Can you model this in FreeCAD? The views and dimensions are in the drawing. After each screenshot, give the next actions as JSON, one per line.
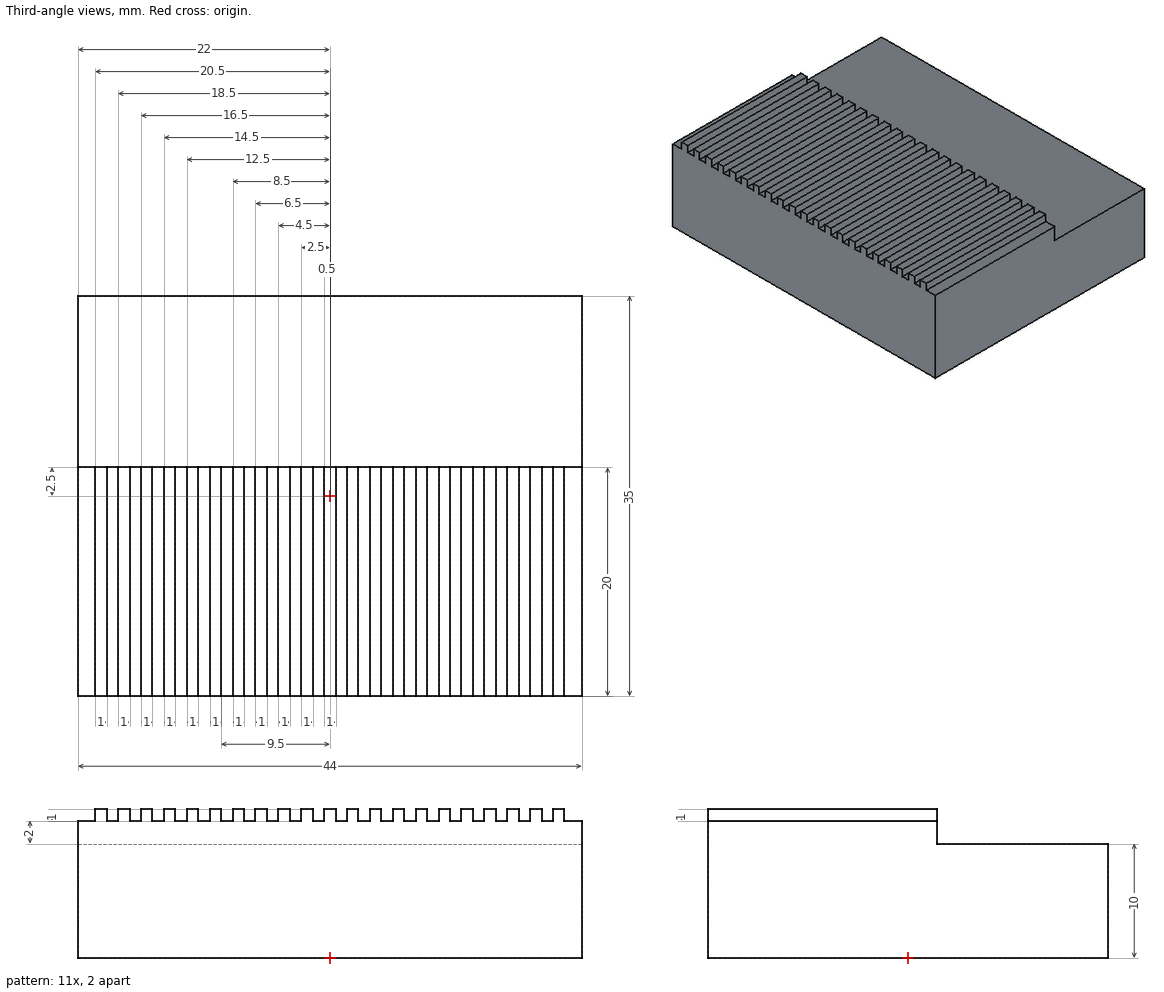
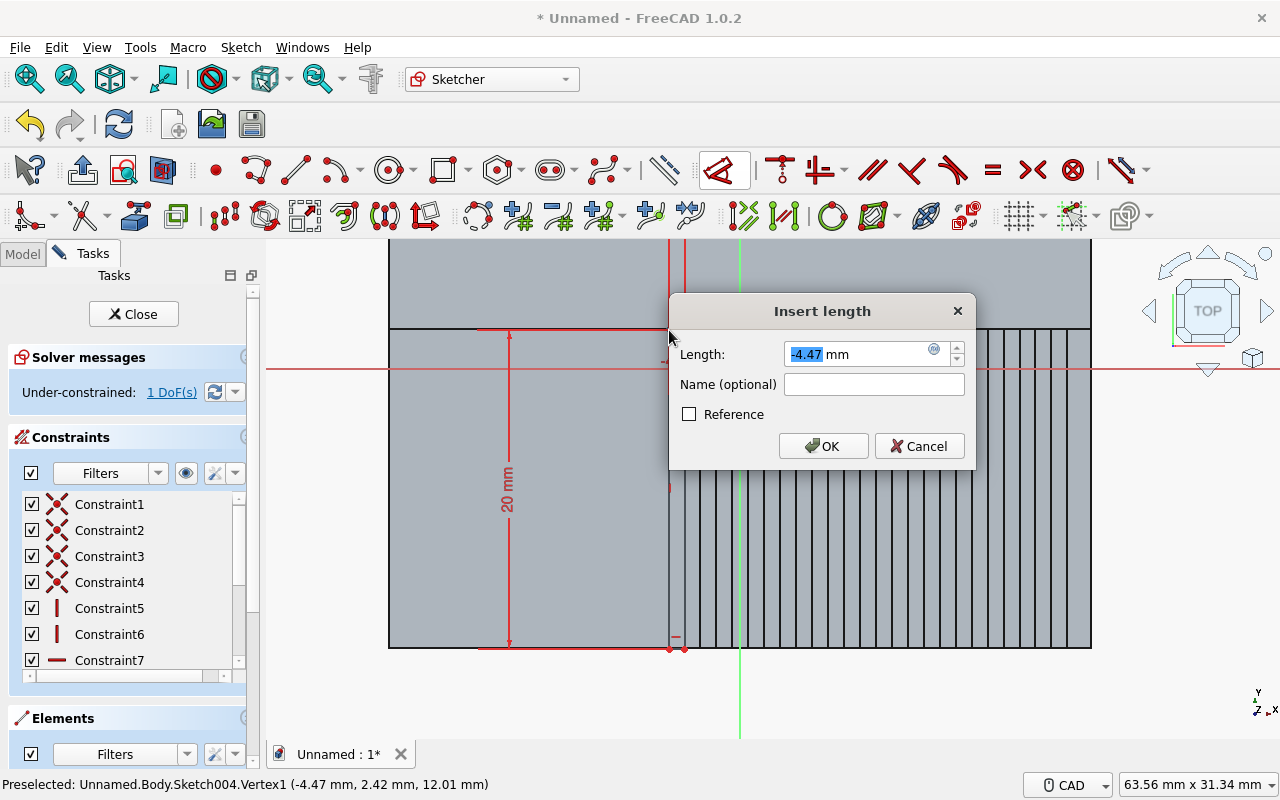
{"action": "type", "text": "-4.5"}
{"action": "key", "text": "Return"}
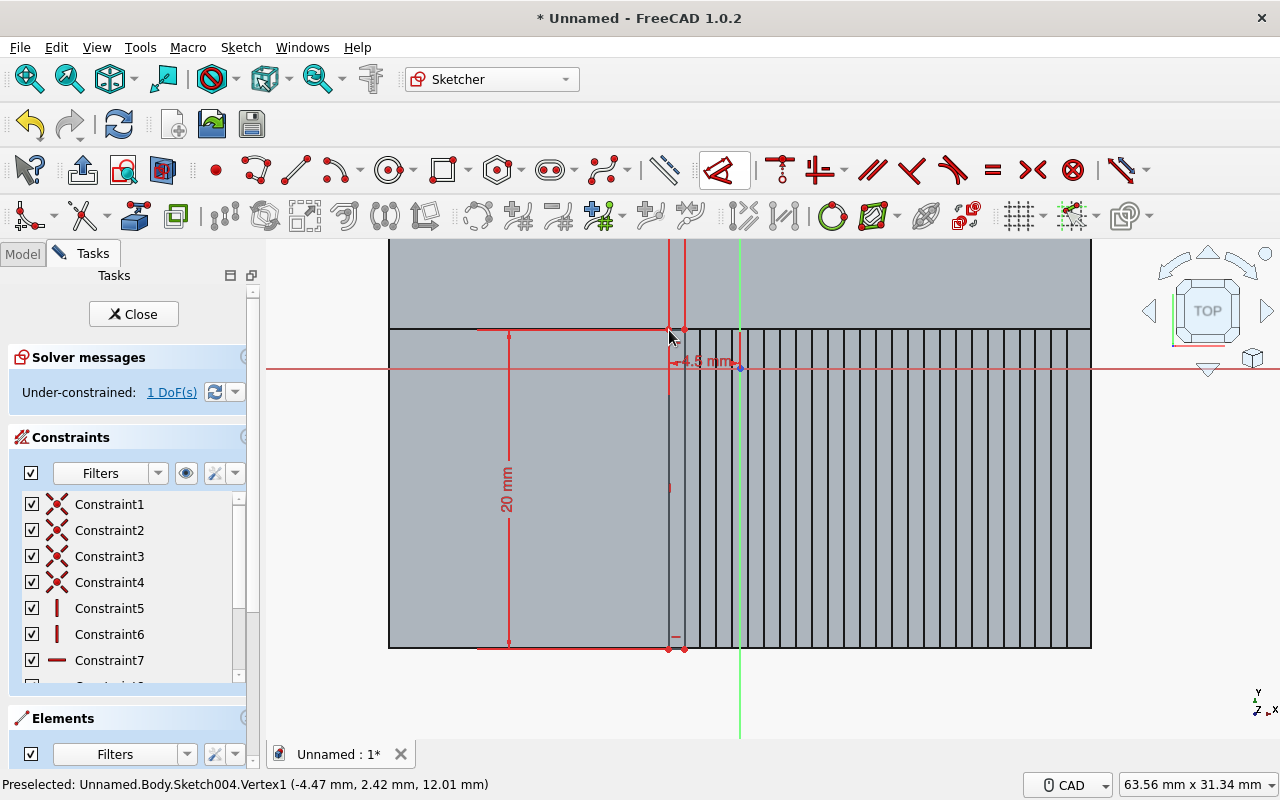
{"action": "left_click", "coordinate": [669, 330]}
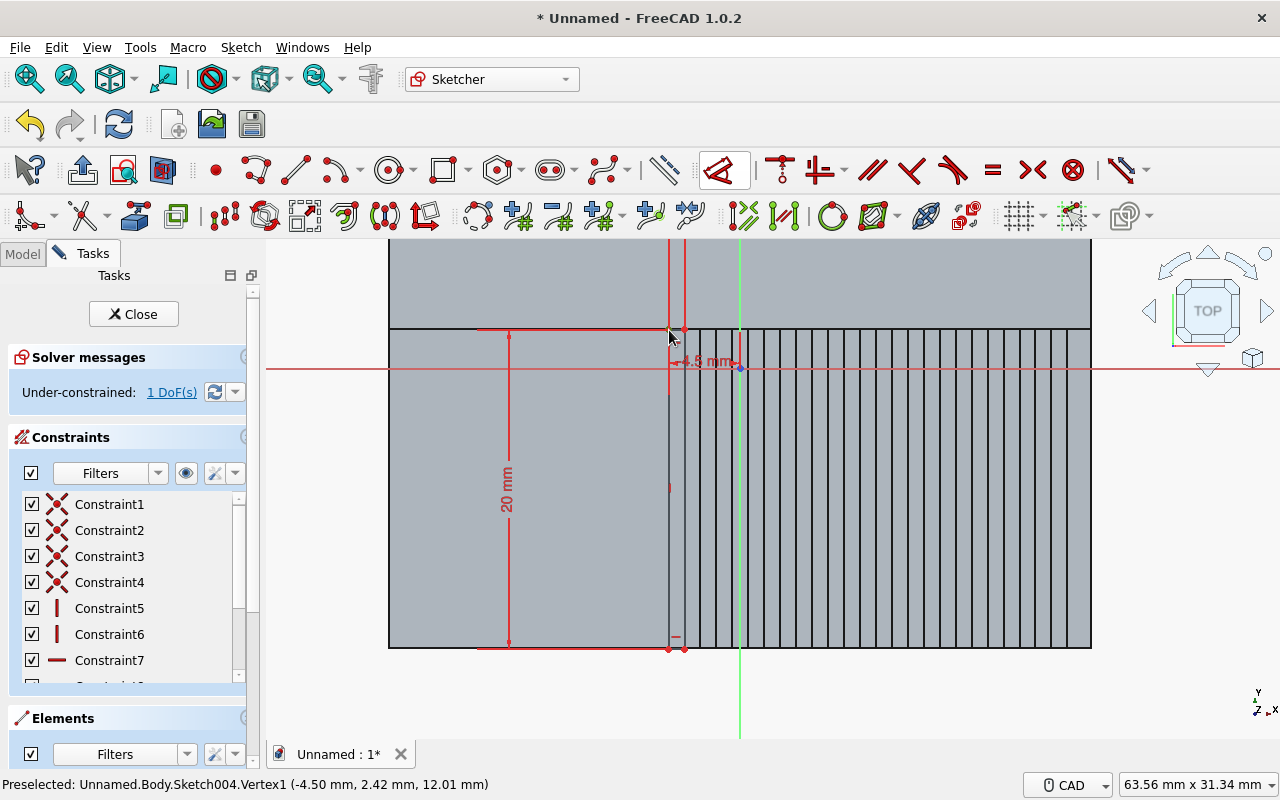
{"action": "key", "text": "i"}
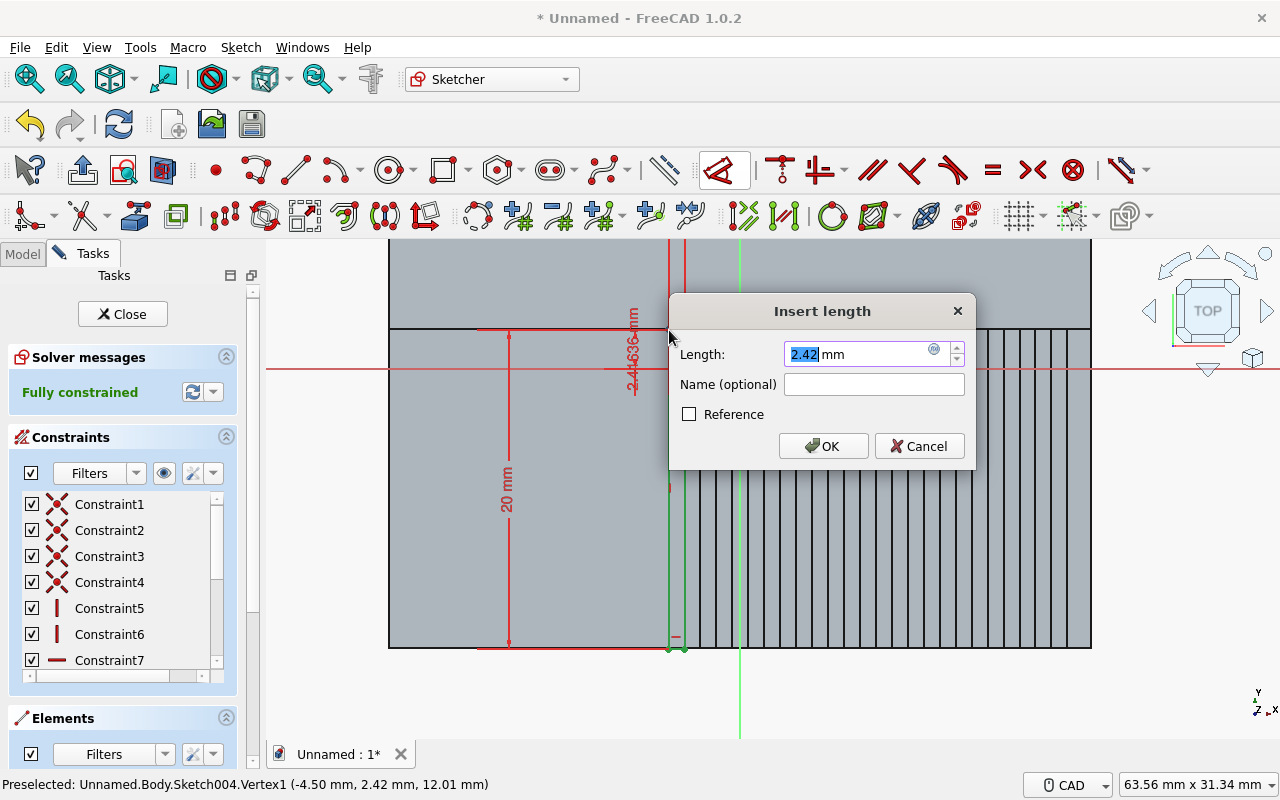
{"action": "type", "text": "2.5"}
{"action": "key", "text": "Return"}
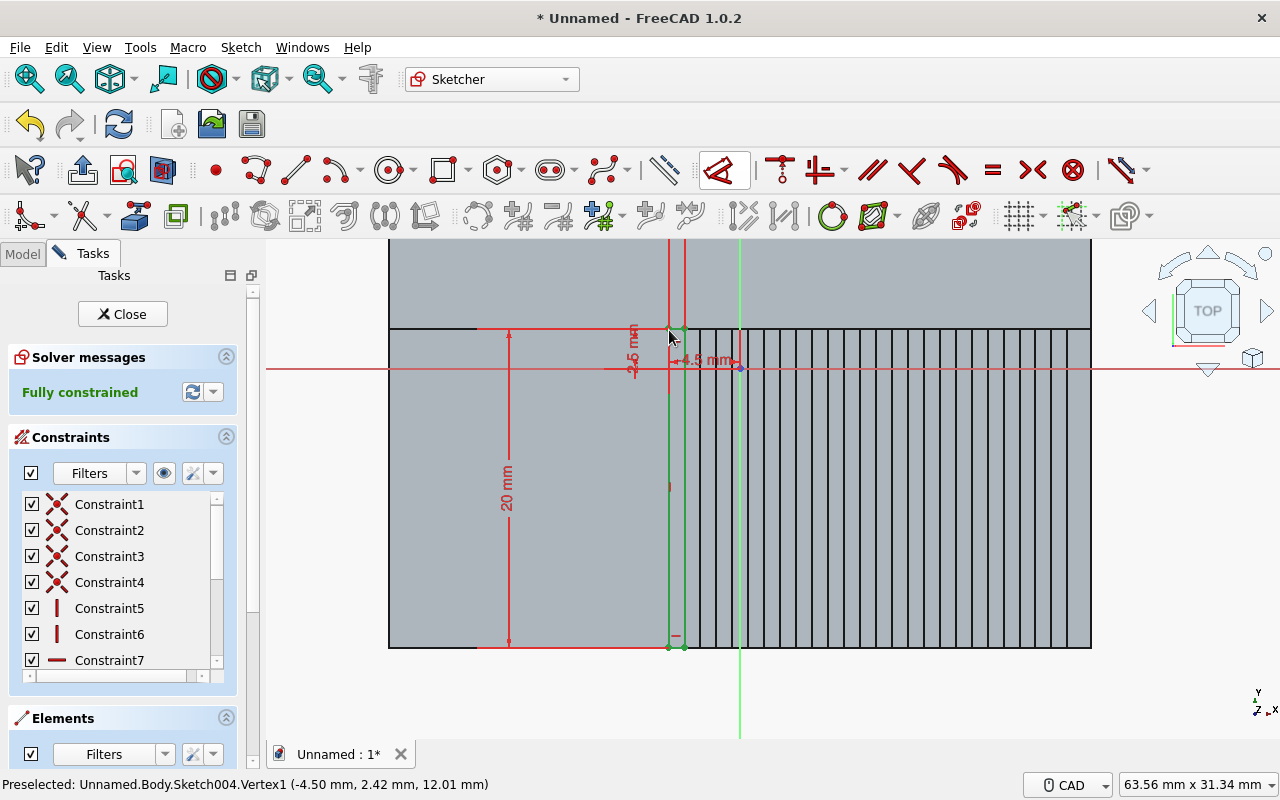
{"action": "left_click", "coordinate": [123, 314]}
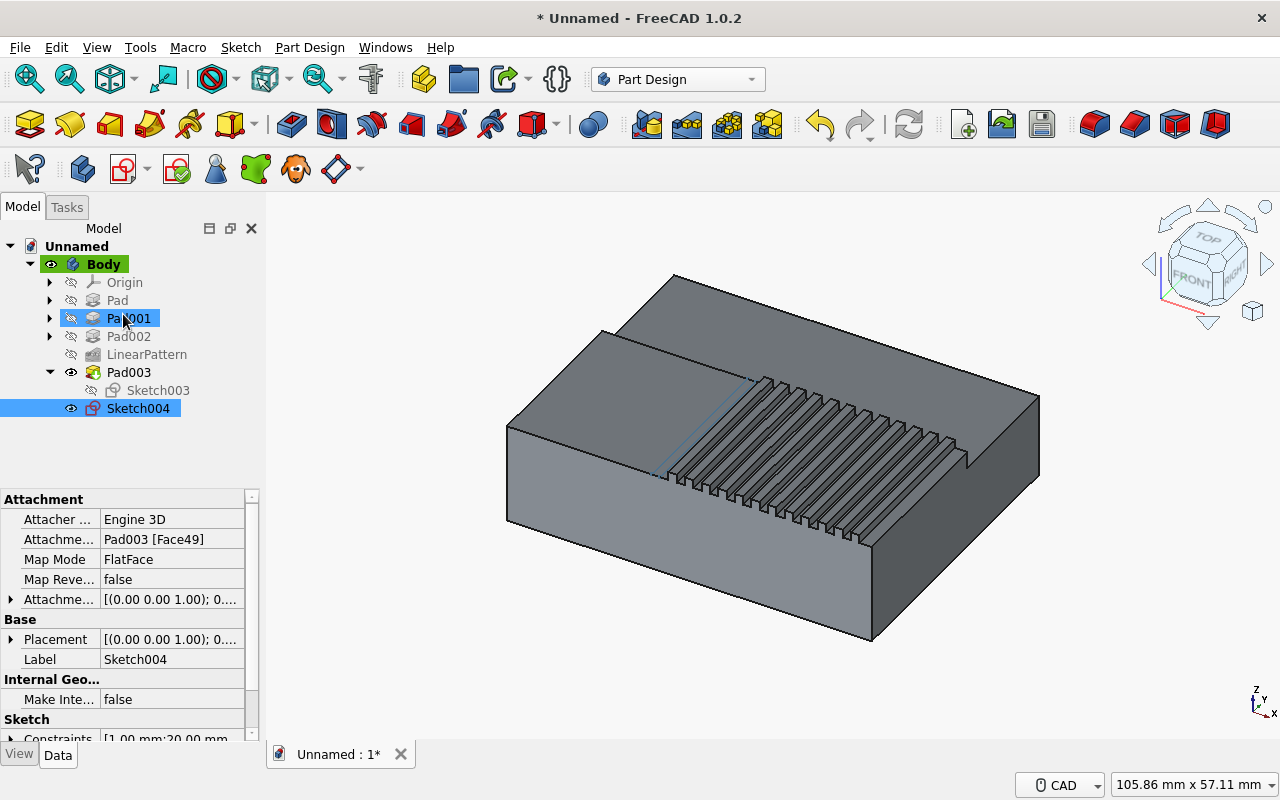
{"action": "left_click", "coordinate": [30, 124]}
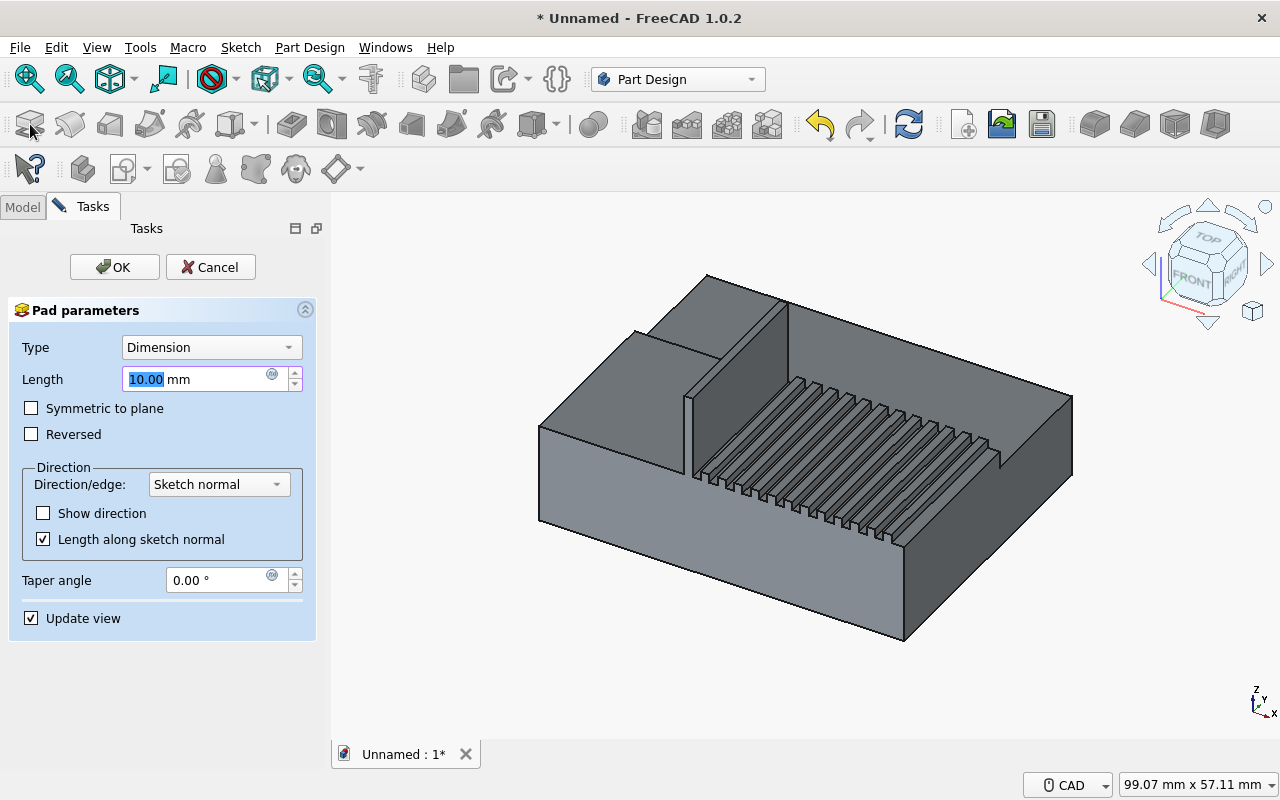
{"action": "type", "text": "1"}
{"action": "key", "text": "Tab"}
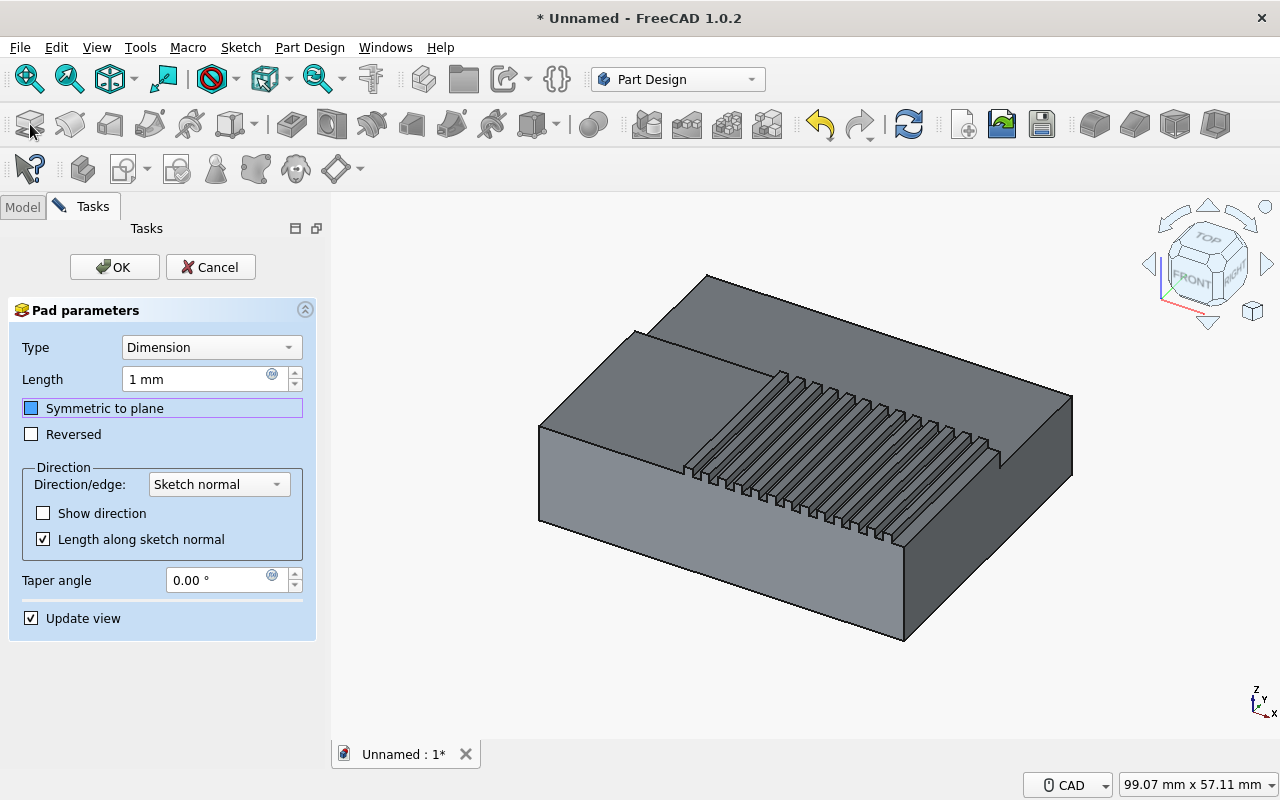
{"action": "left_click", "coordinate": [115, 267]}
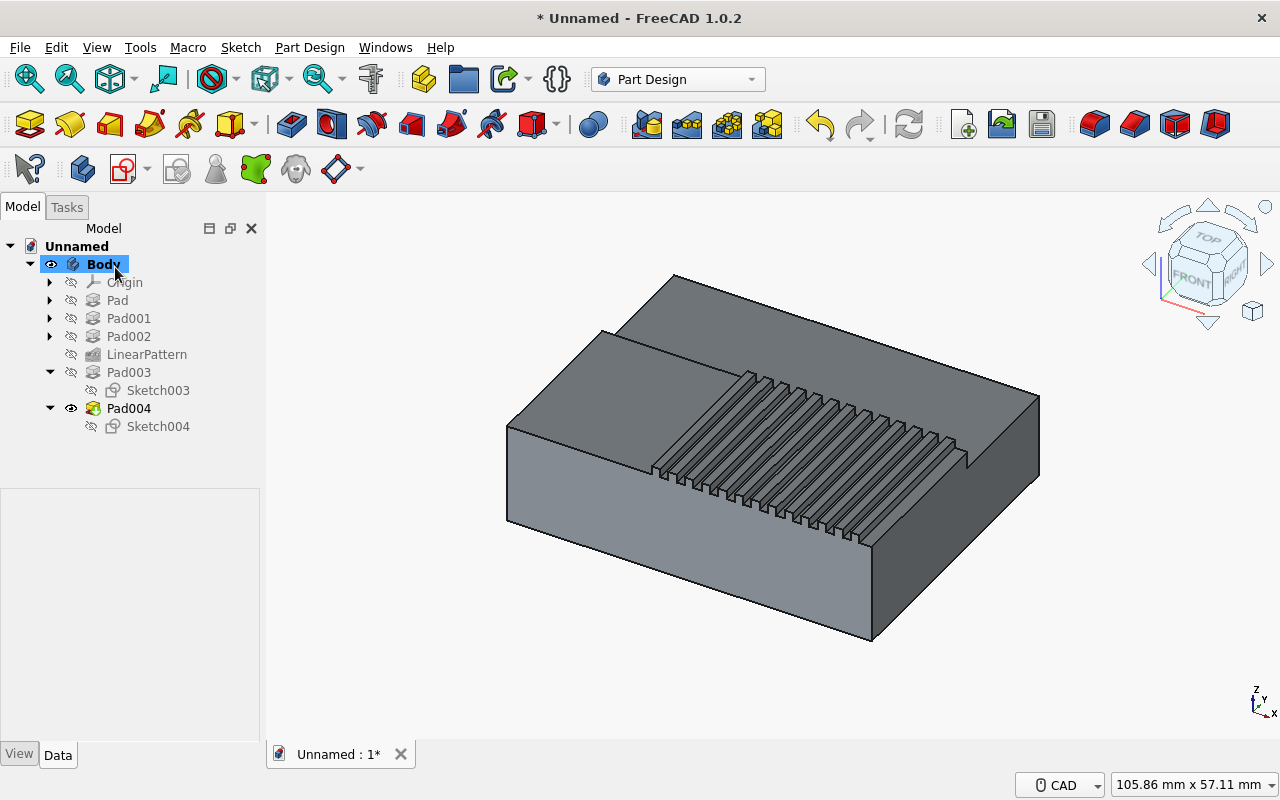
{"action": "left_click", "coordinate": [627, 402]}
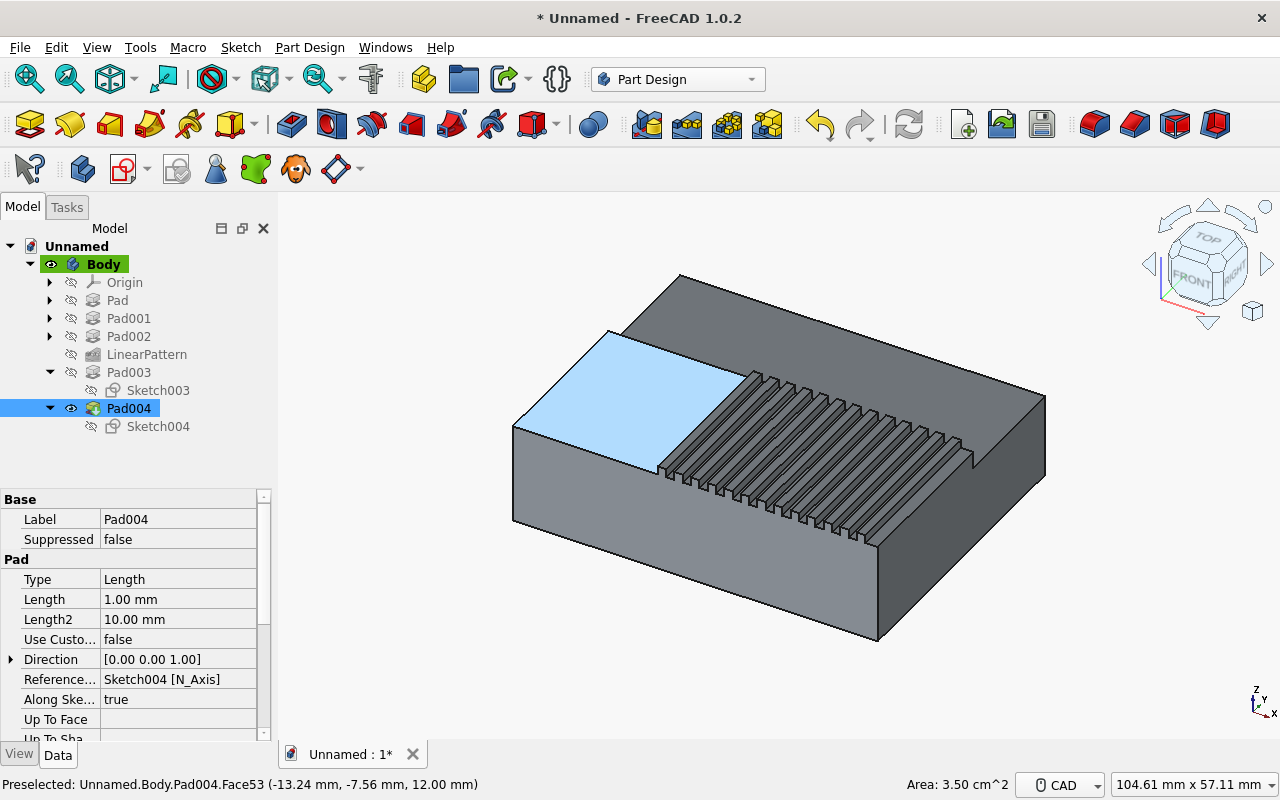
{"action": "left_click", "coordinate": [124, 170]}